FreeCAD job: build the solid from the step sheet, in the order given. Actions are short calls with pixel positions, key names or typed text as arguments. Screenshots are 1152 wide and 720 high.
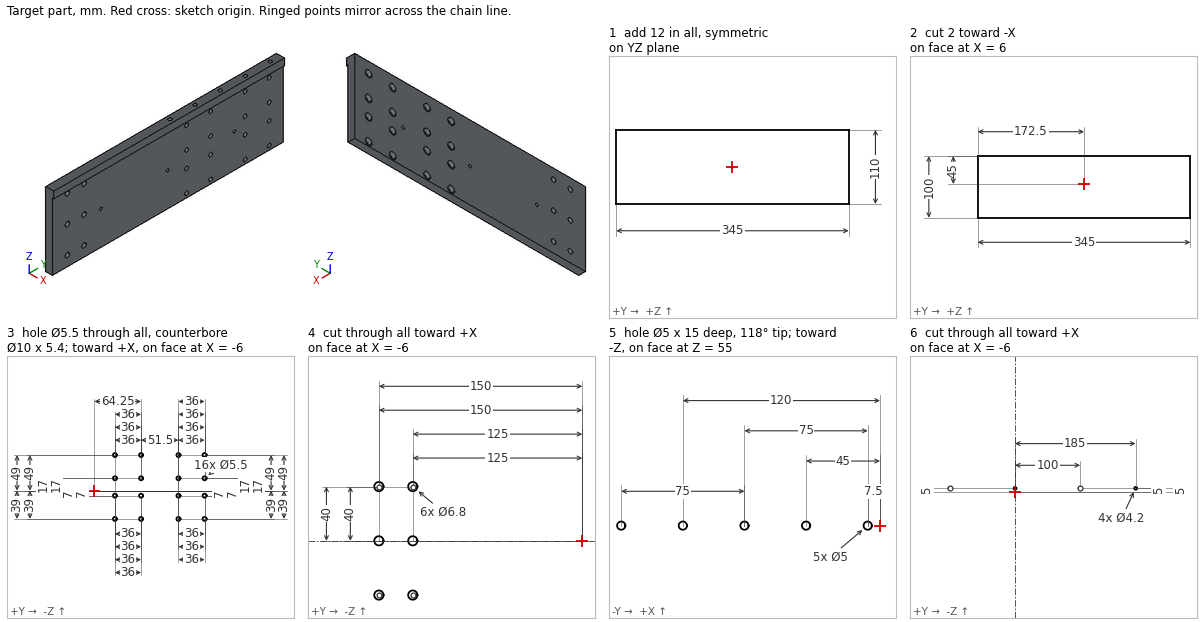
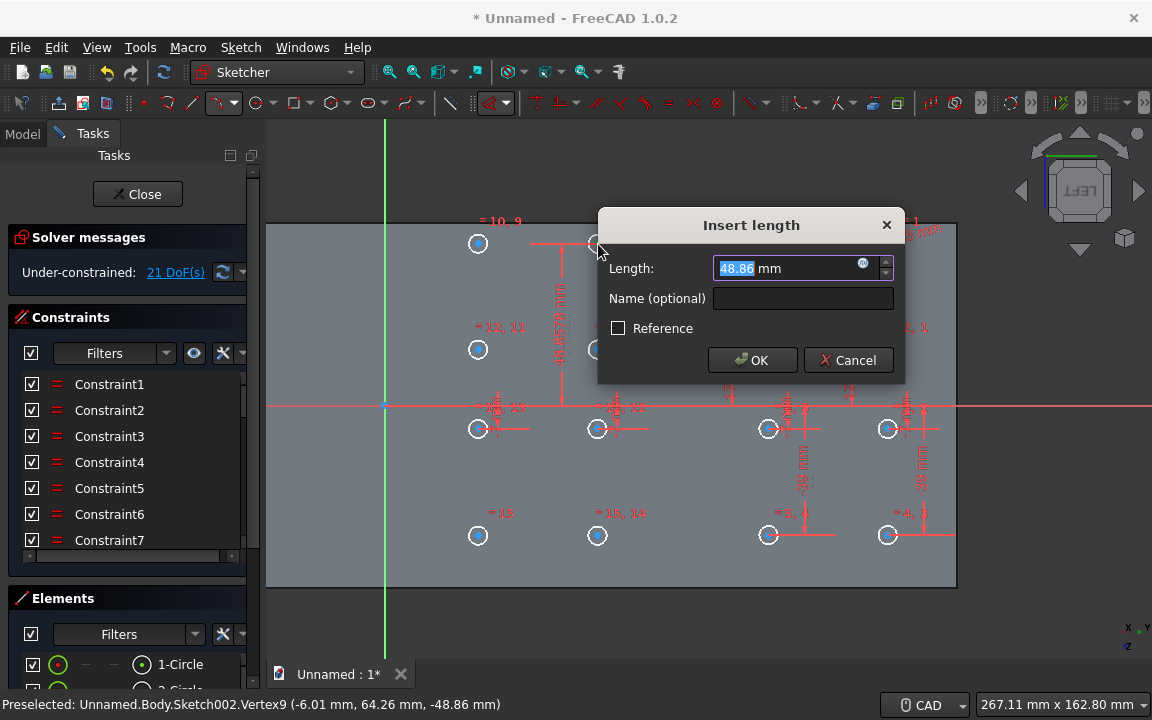
text(49)
key(Return)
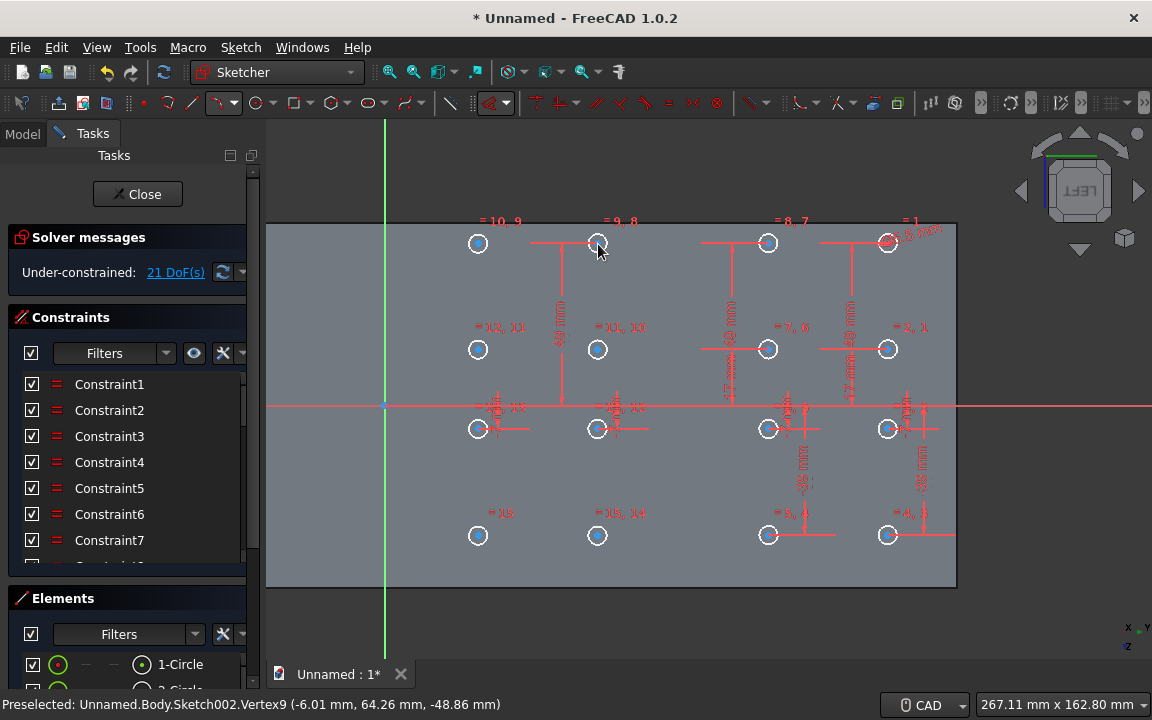
click(478, 244)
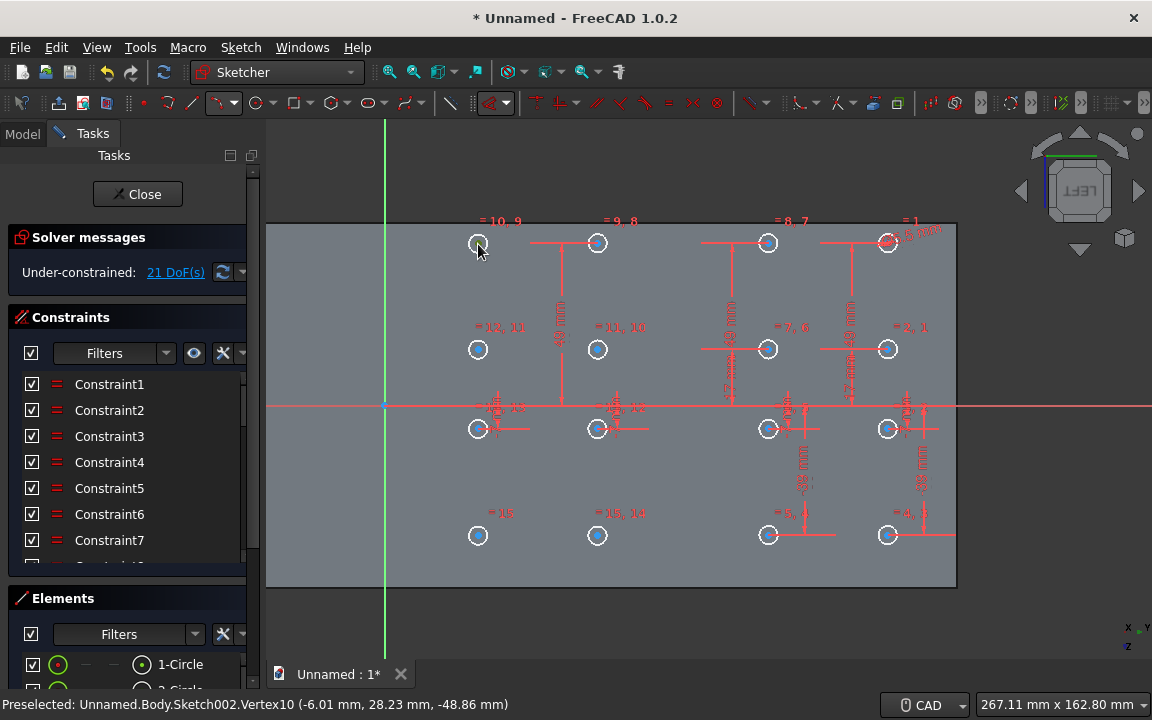
click(508, 104)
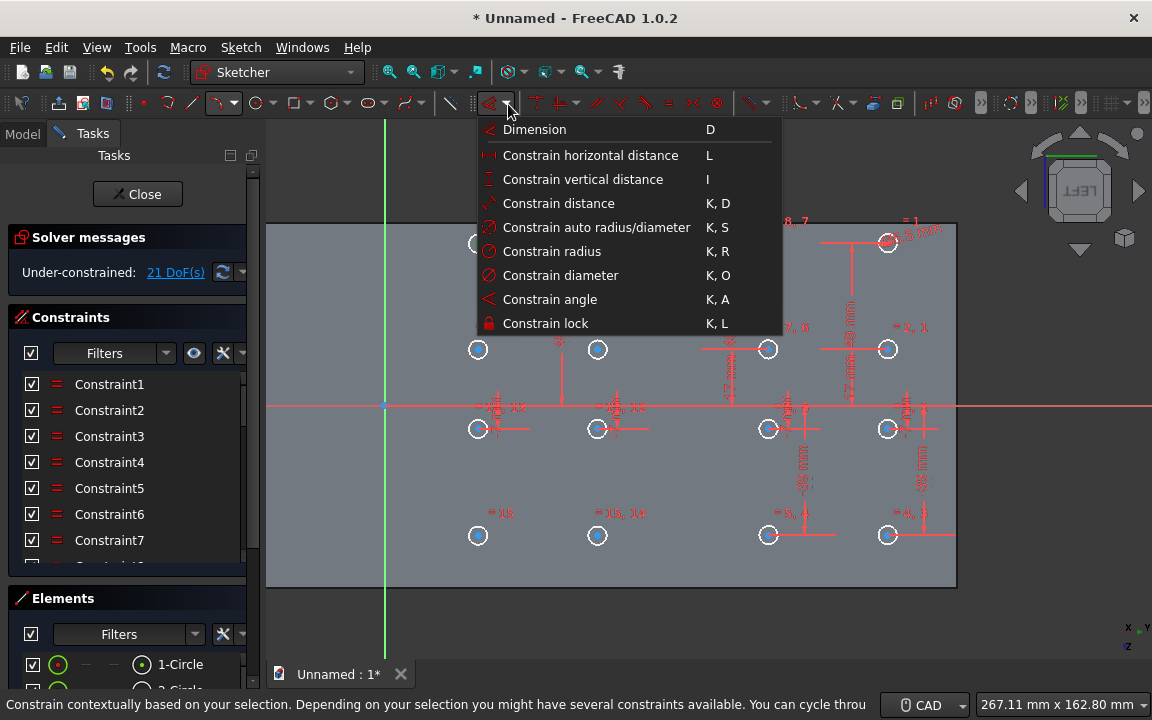
click(630, 179)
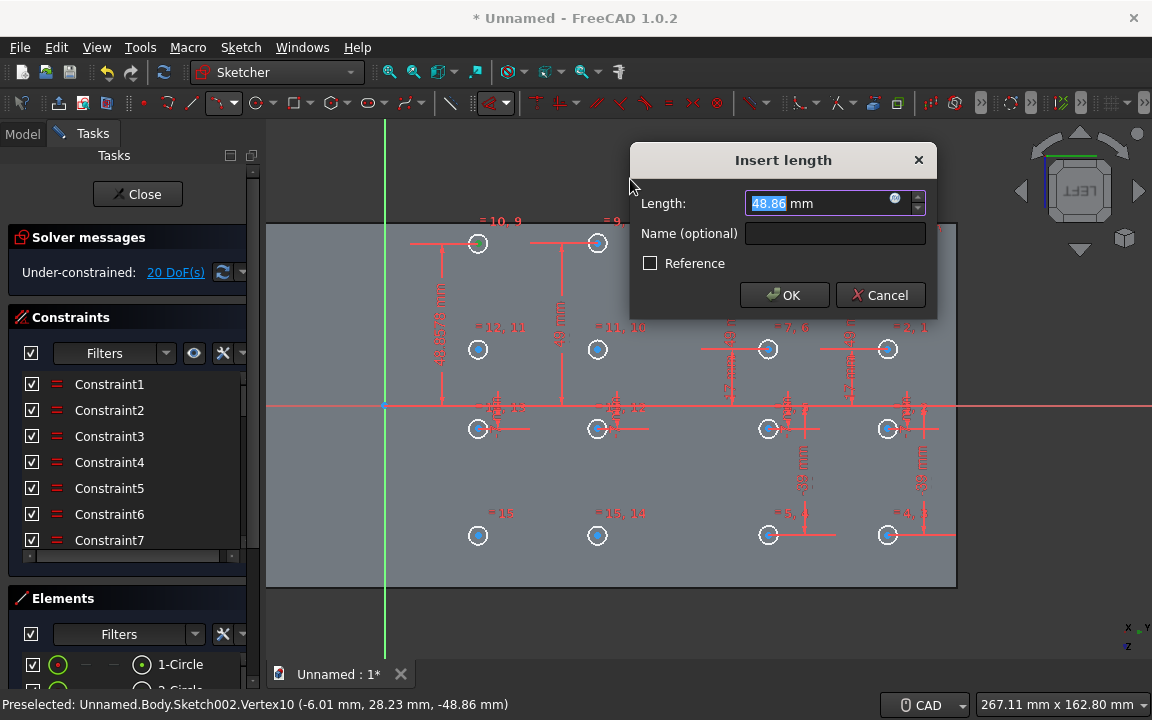
text(49)
key(Return)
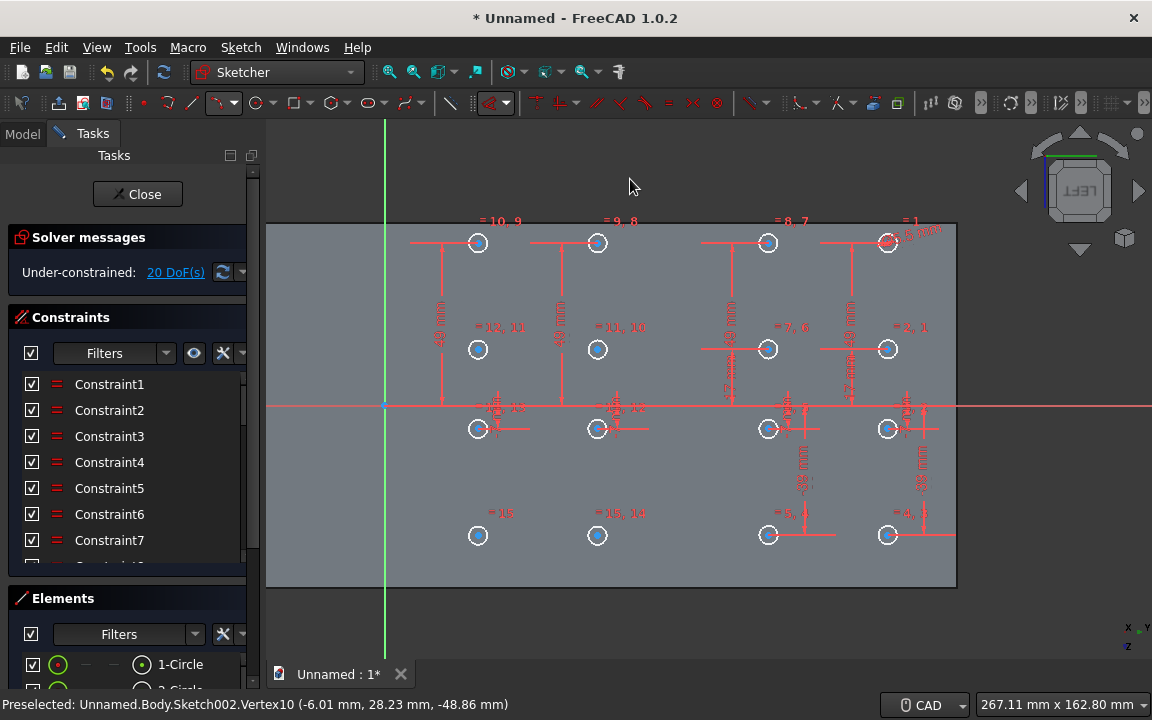
click(598, 350)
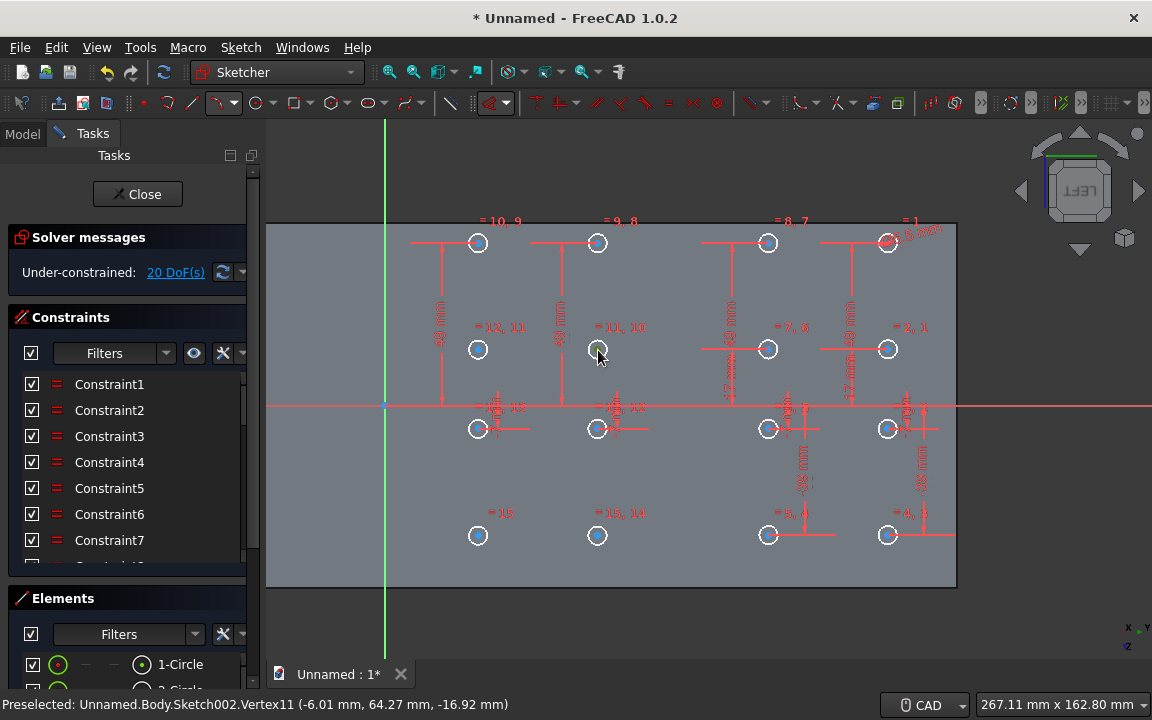
click(508, 104)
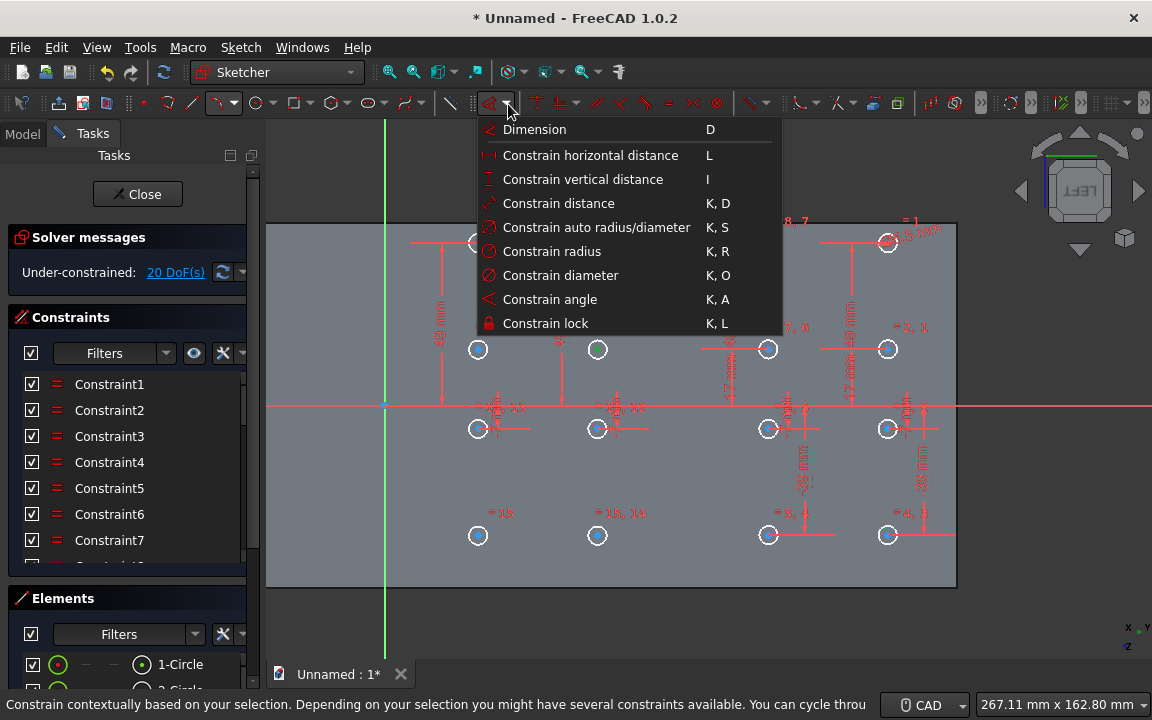
click(630, 179)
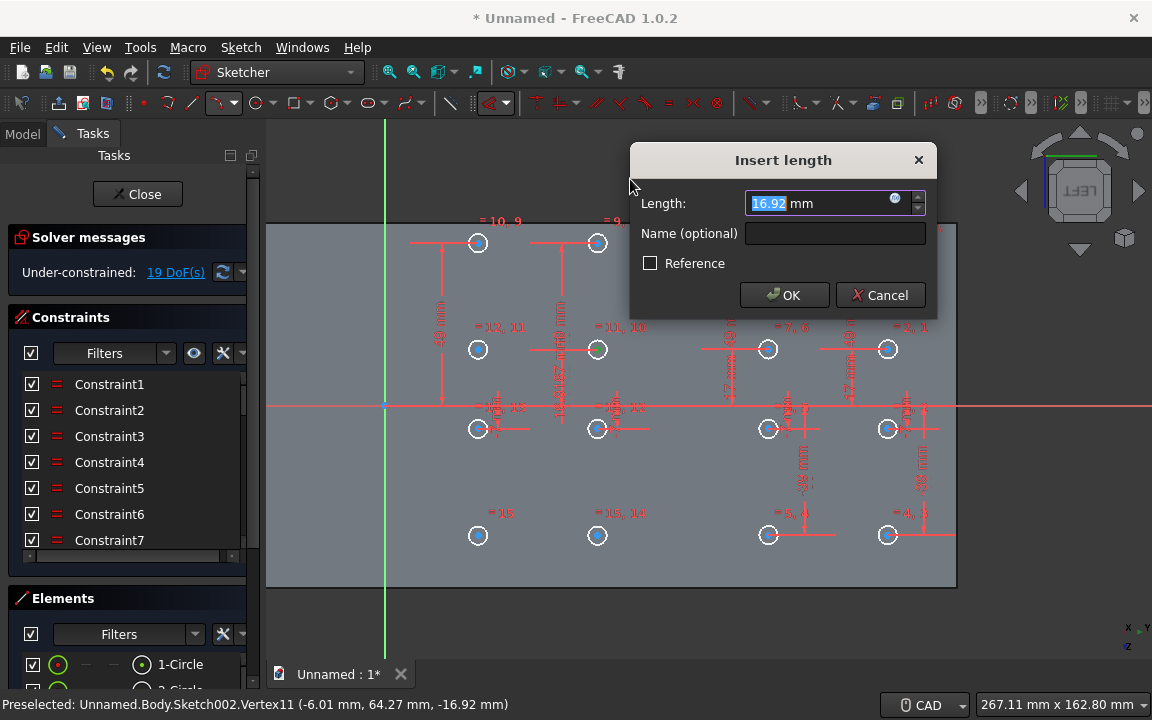
text(17)
key(Return)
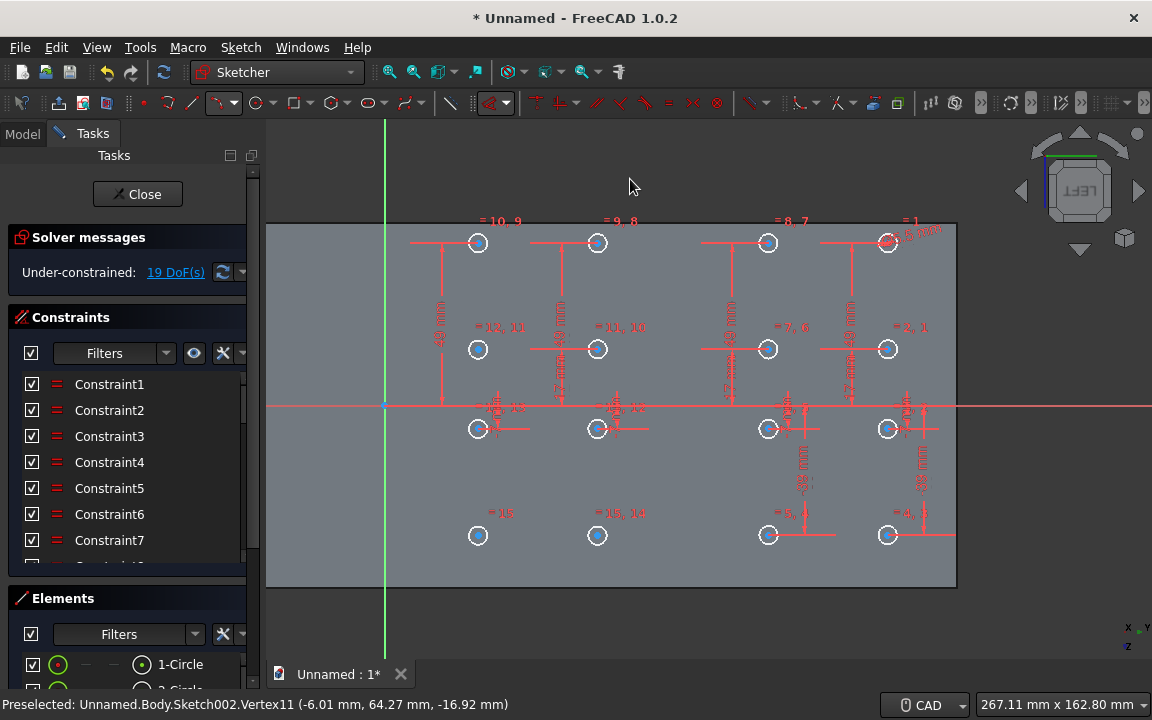
click(478, 350)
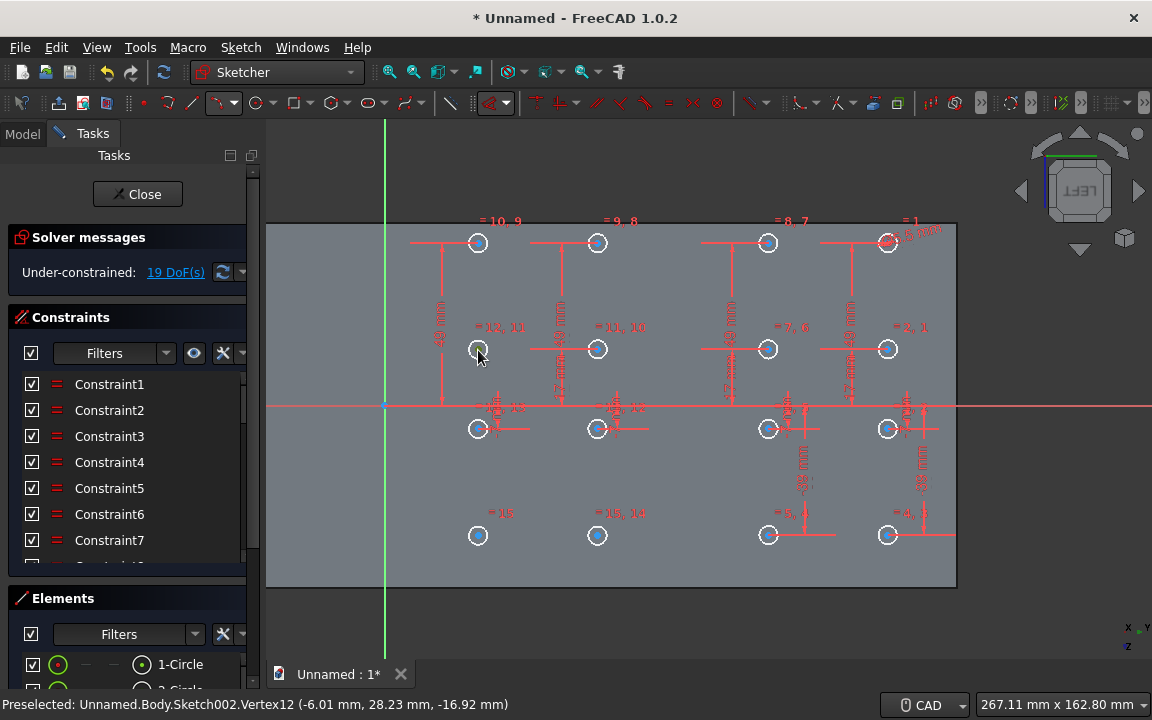
click(508, 104)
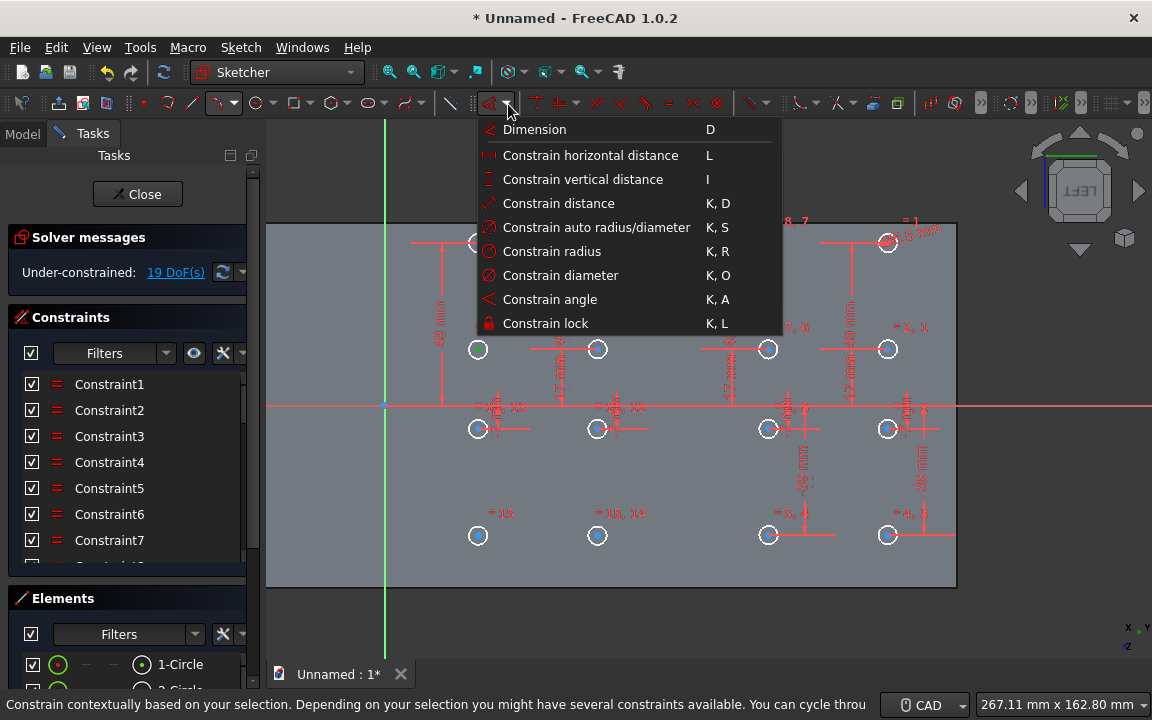
click(630, 179)